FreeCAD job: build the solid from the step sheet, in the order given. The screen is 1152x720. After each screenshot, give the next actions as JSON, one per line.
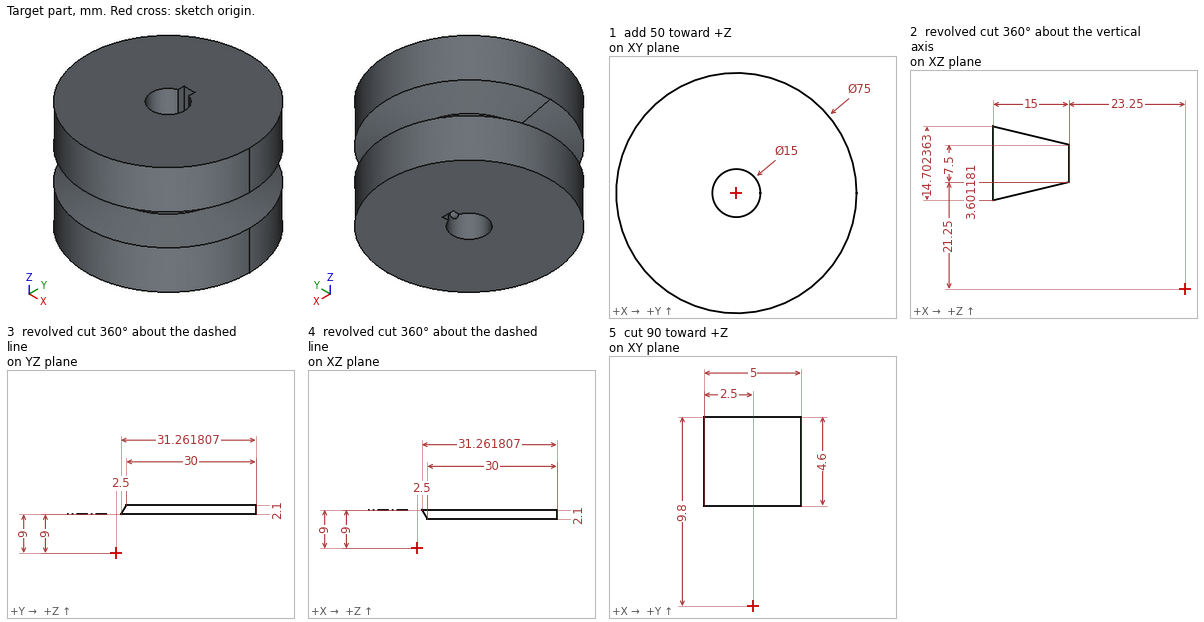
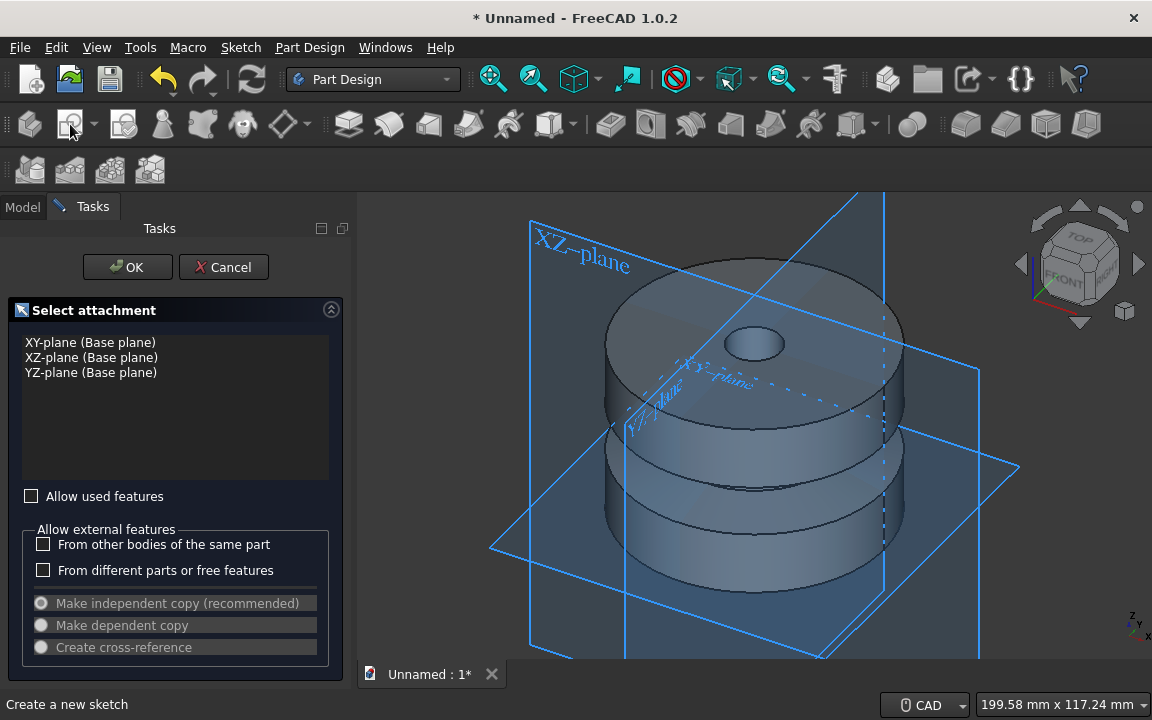
{"action": "left_click", "coordinate": [82, 358]}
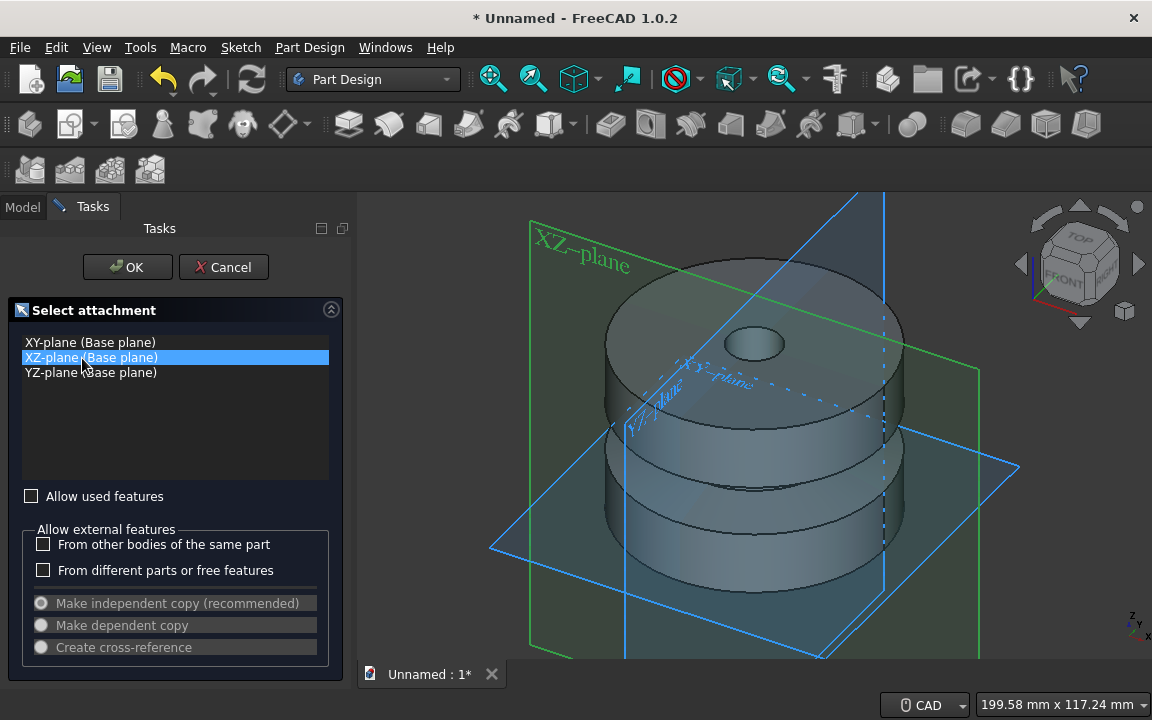
{"action": "left_click", "coordinate": [128, 267]}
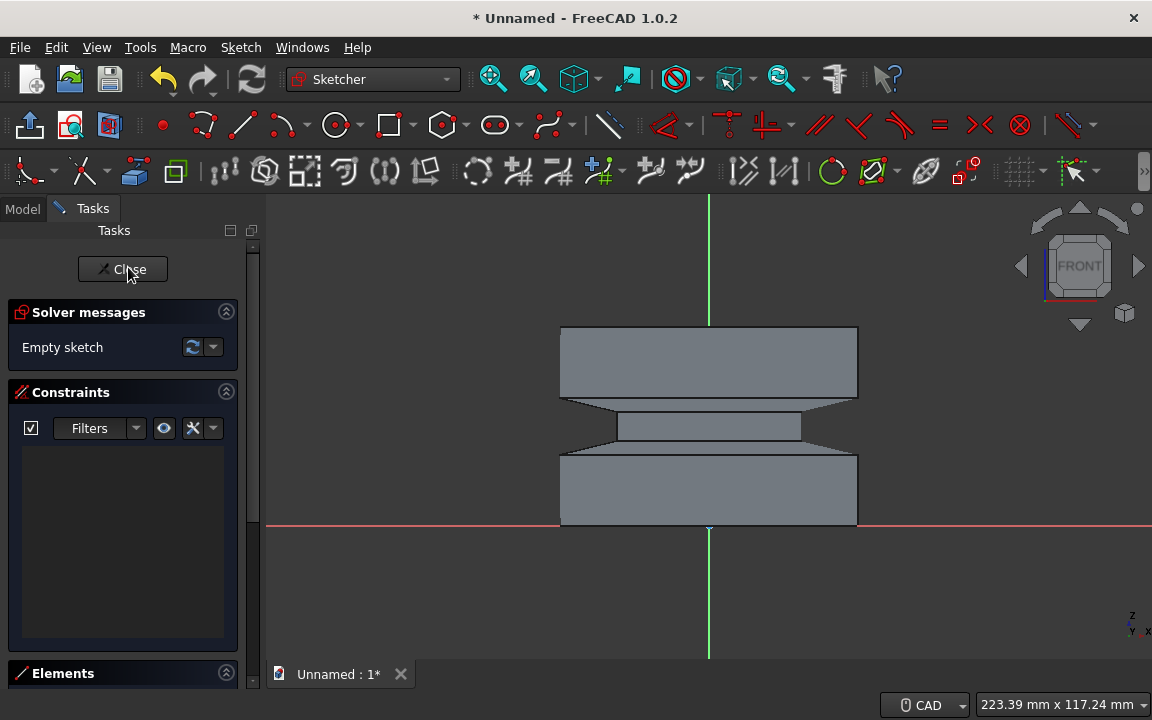
{"action": "left_click", "coordinate": [110, 126]}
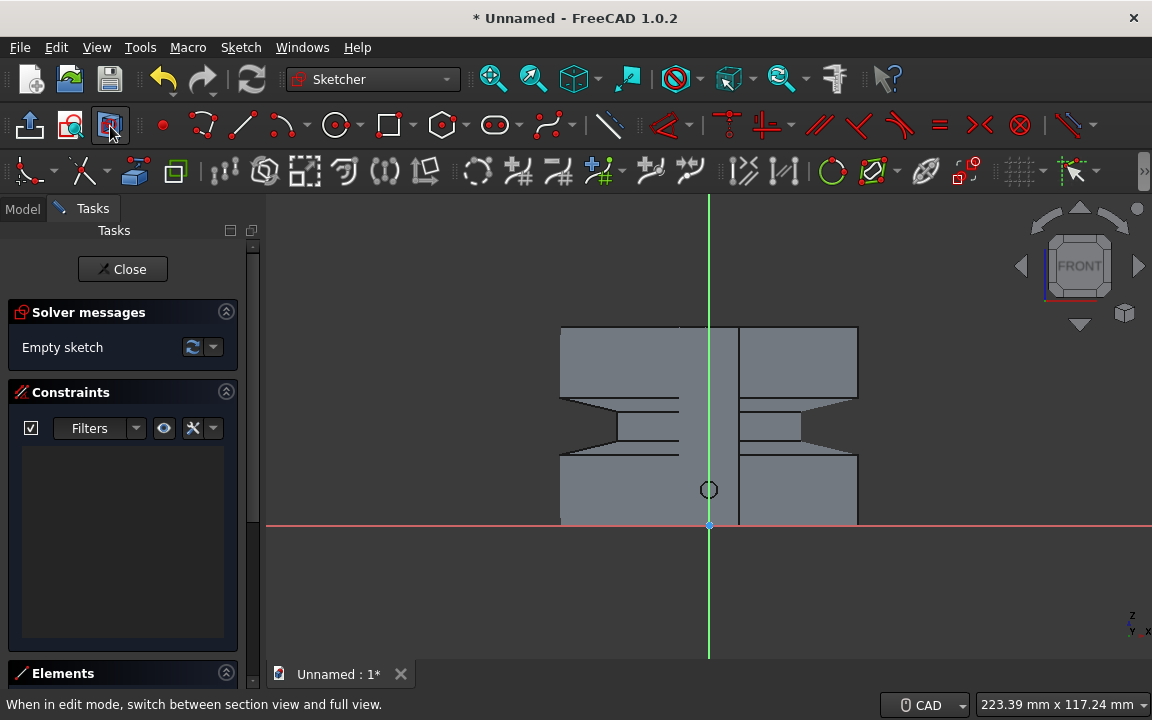
{"action": "scroll", "coordinate": [815, 555], "scroll_direction": "up", "scroll_amount": 5}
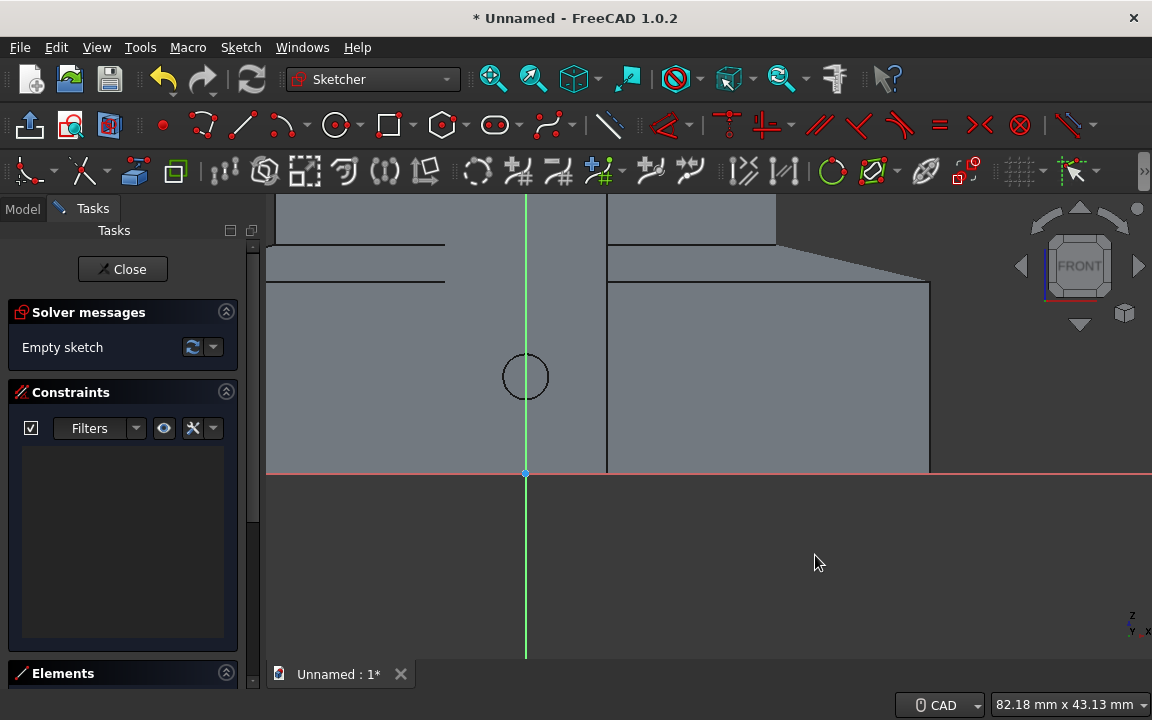
{"action": "left_click", "coordinate": [204, 126]}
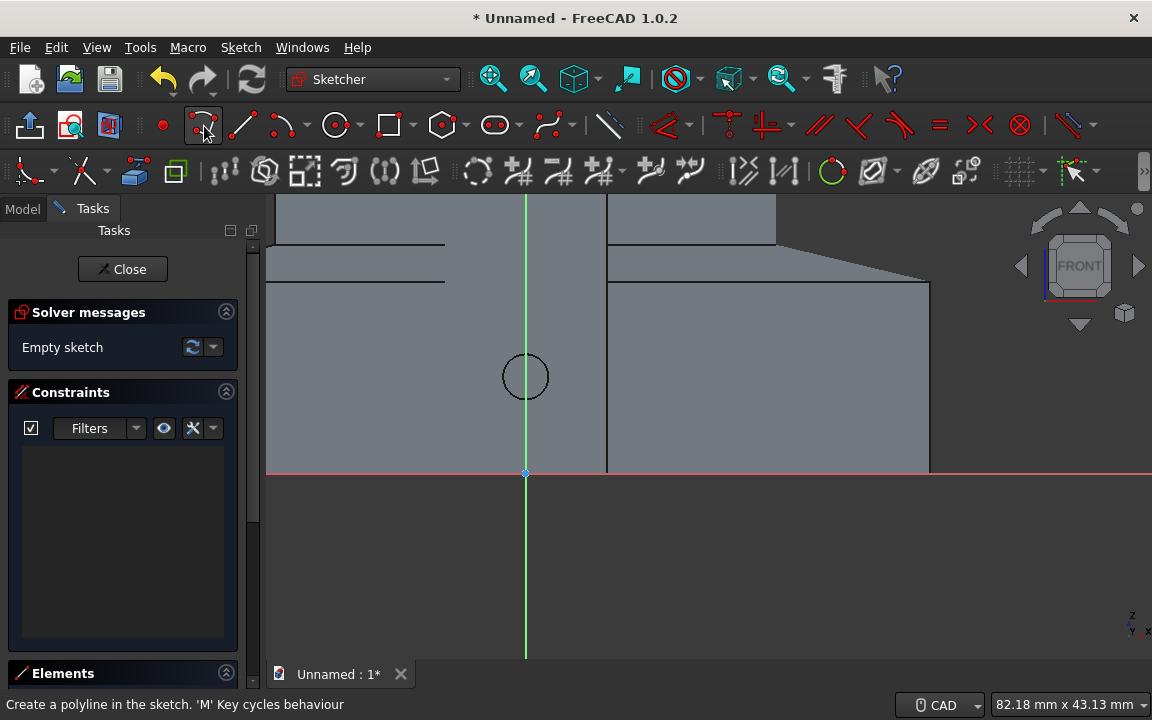
{"action": "left_click", "coordinate": [553, 400]}
{"action": "left_click", "coordinate": [539, 377]}
{"action": "left_click", "coordinate": [876, 377]}
{"action": "left_click", "coordinate": [876, 400]}
{"action": "left_click", "coordinate": [553, 401]}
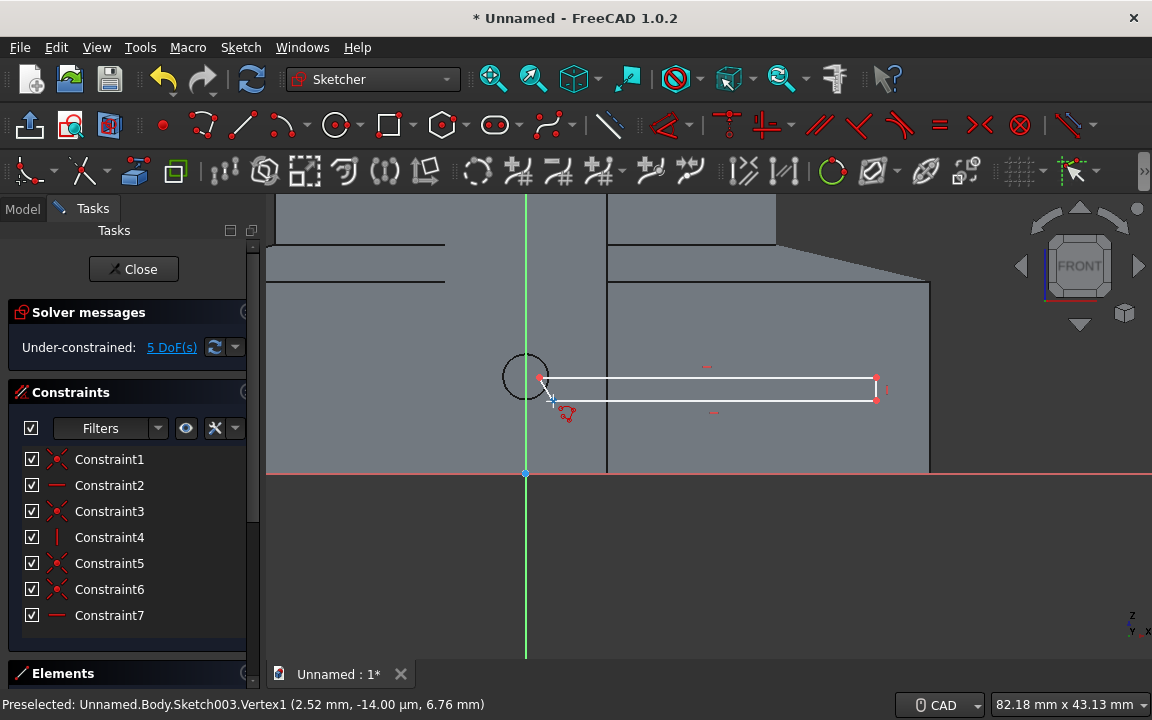
{"action": "left_click", "coordinate": [244, 126]}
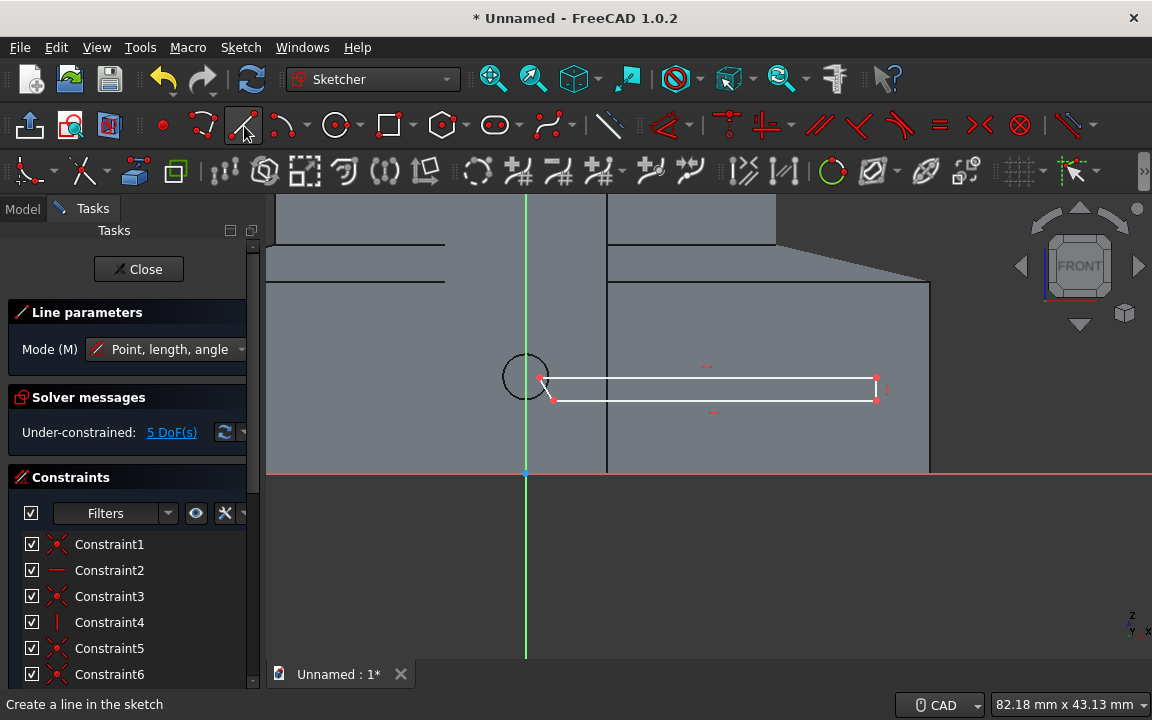
{"action": "left_click", "coordinate": [505, 377]}
{"action": "left_click", "coordinate": [404, 377]}
{"action": "key", "text": "Escape"}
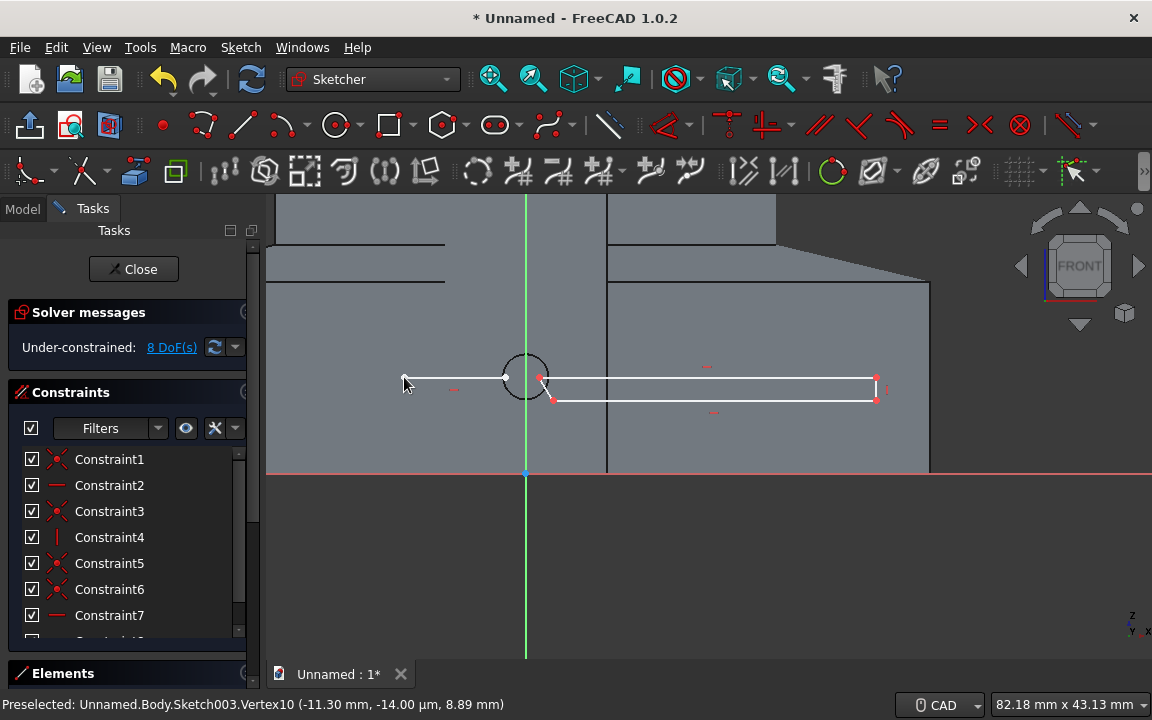
{"action": "left_click", "coordinate": [475, 378]}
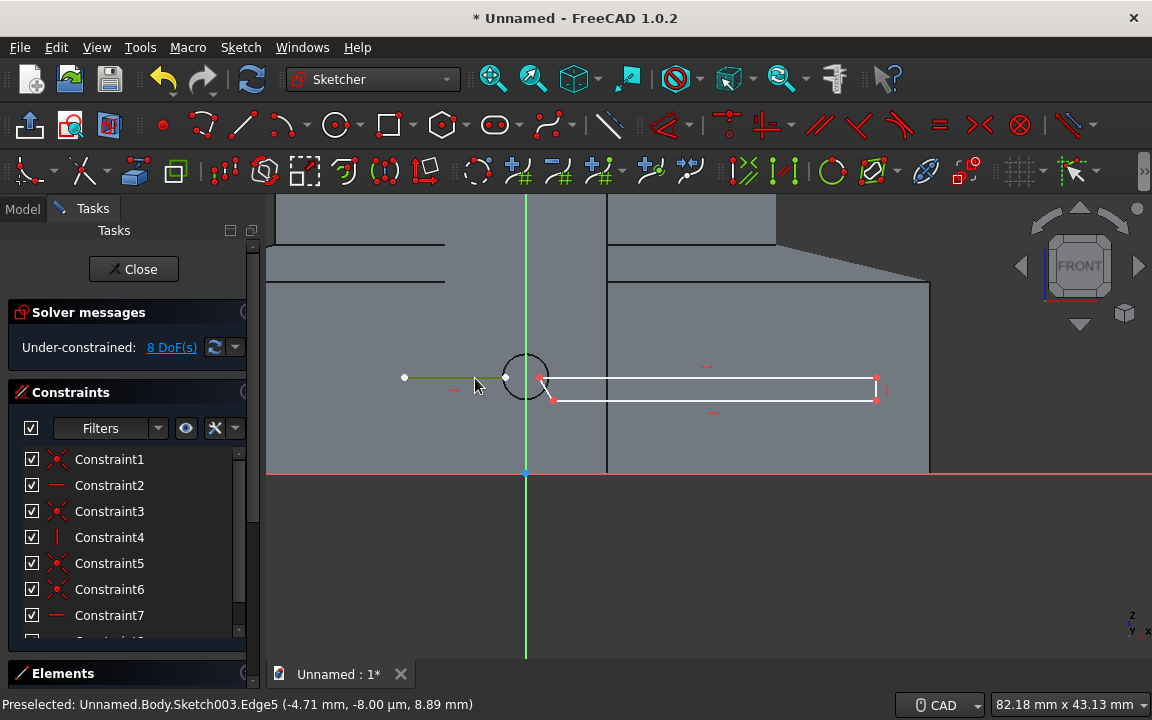
{"action": "left_click", "coordinate": [610, 126]}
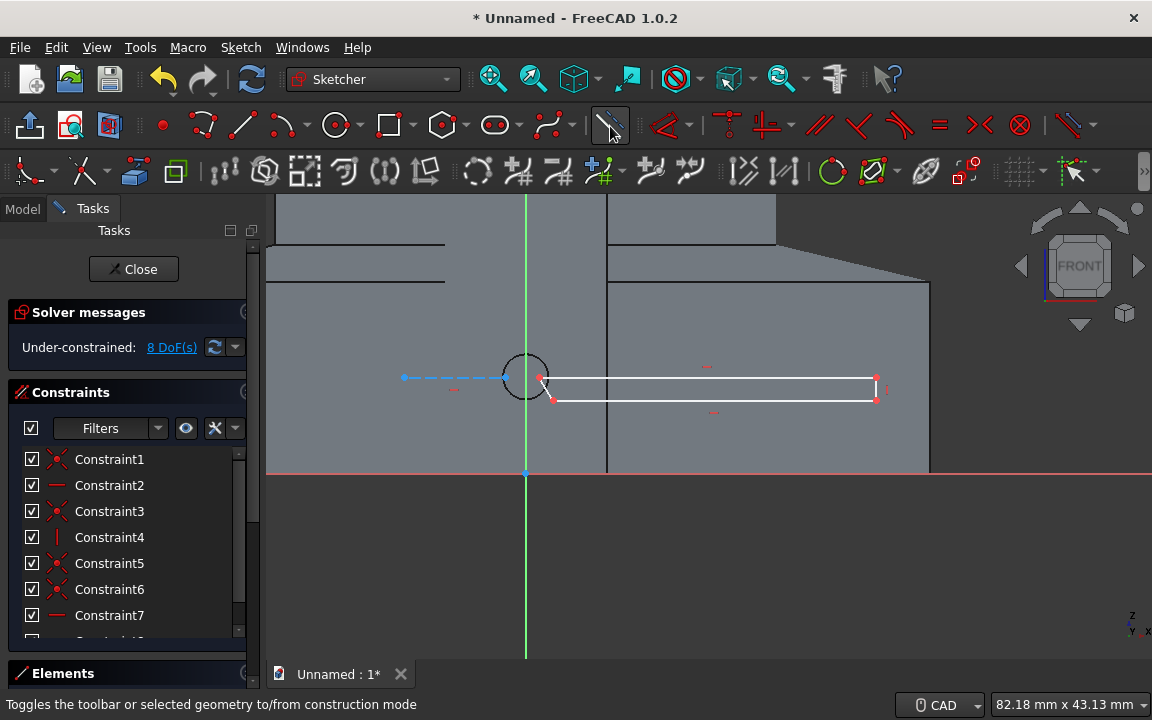
{"action": "left_click", "coordinate": [664, 126]}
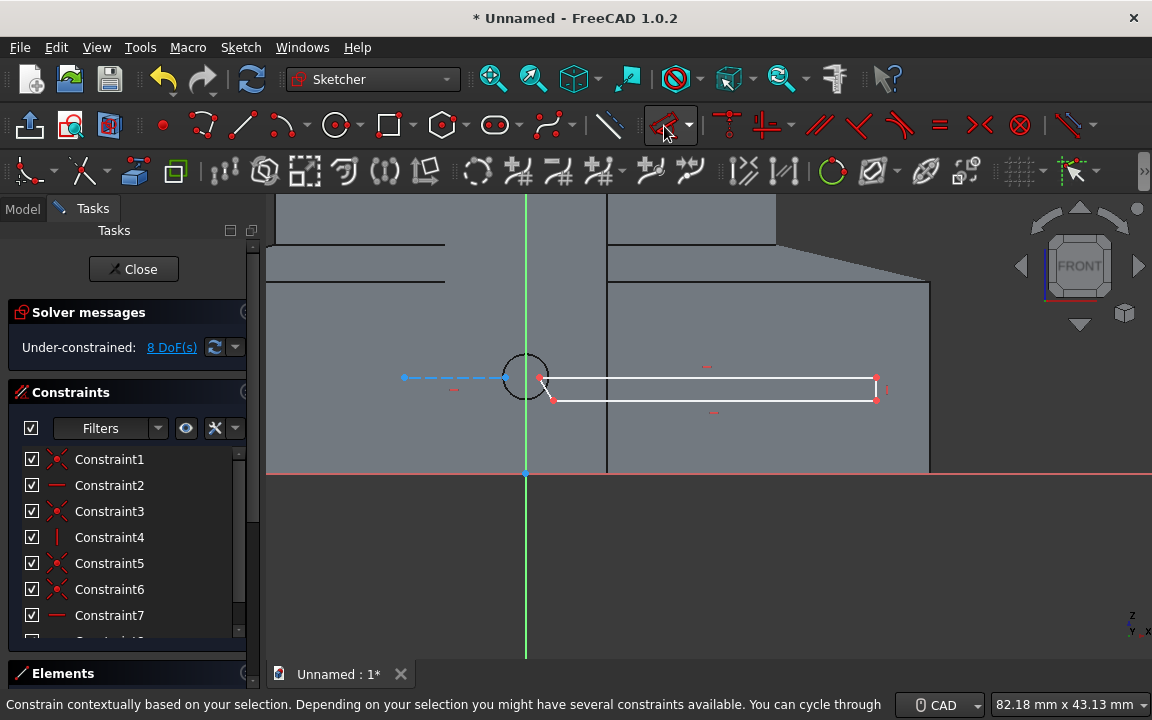
{"action": "left_click", "coordinate": [779, 401]}
{"action": "left_click", "coordinate": [715, 435]}